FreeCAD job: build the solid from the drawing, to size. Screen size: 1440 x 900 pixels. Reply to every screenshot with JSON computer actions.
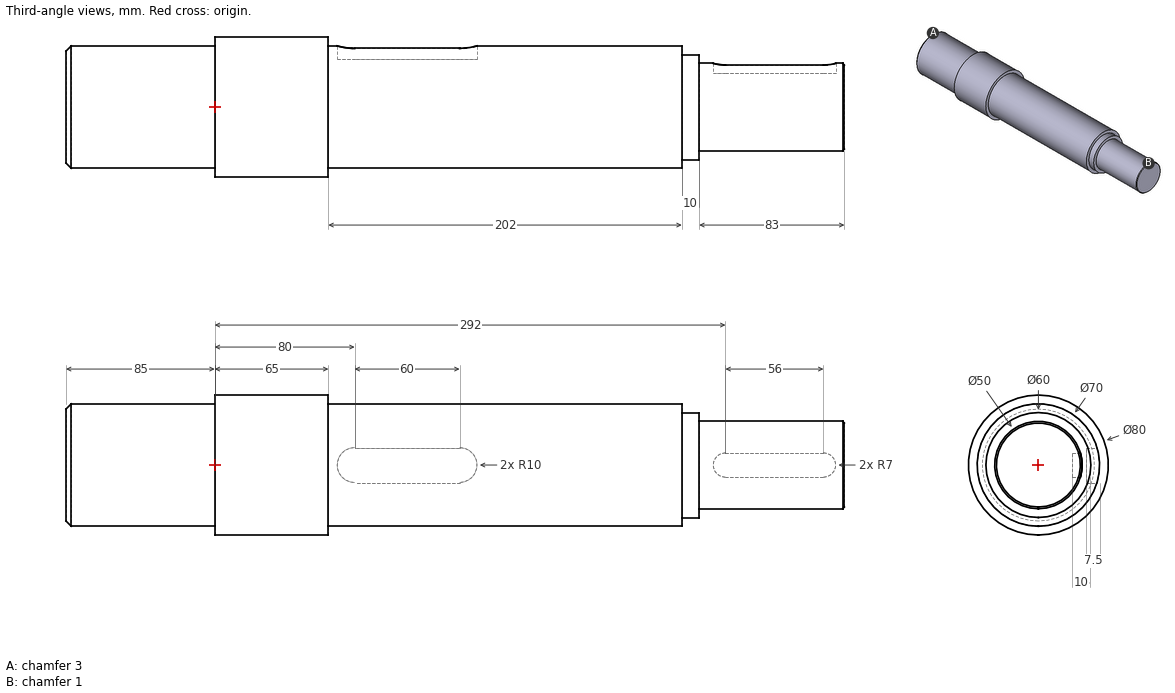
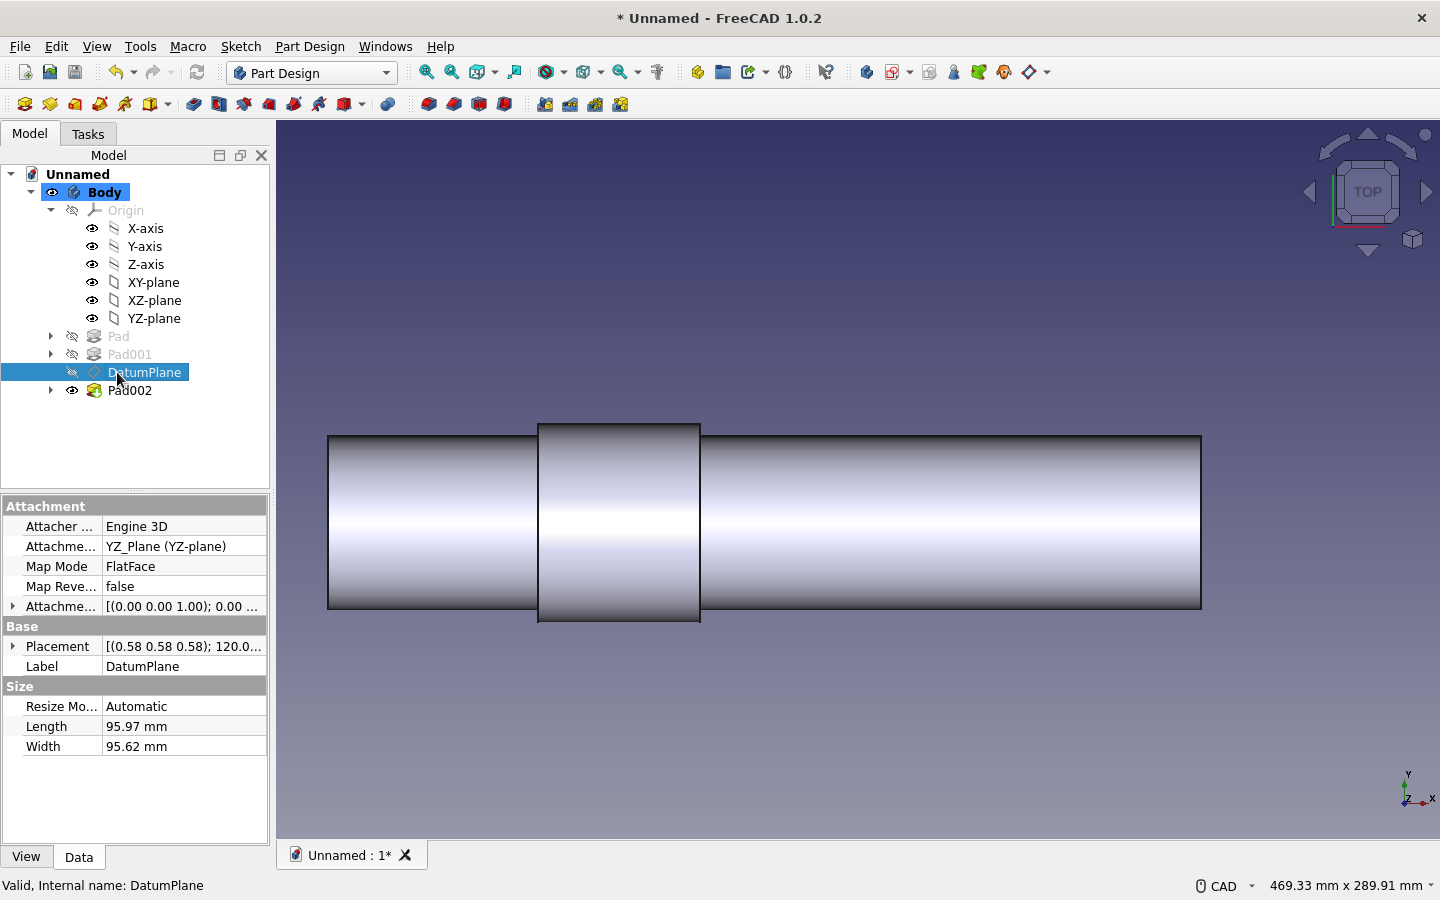
{"action": "left_click", "coordinate": [328, 592]}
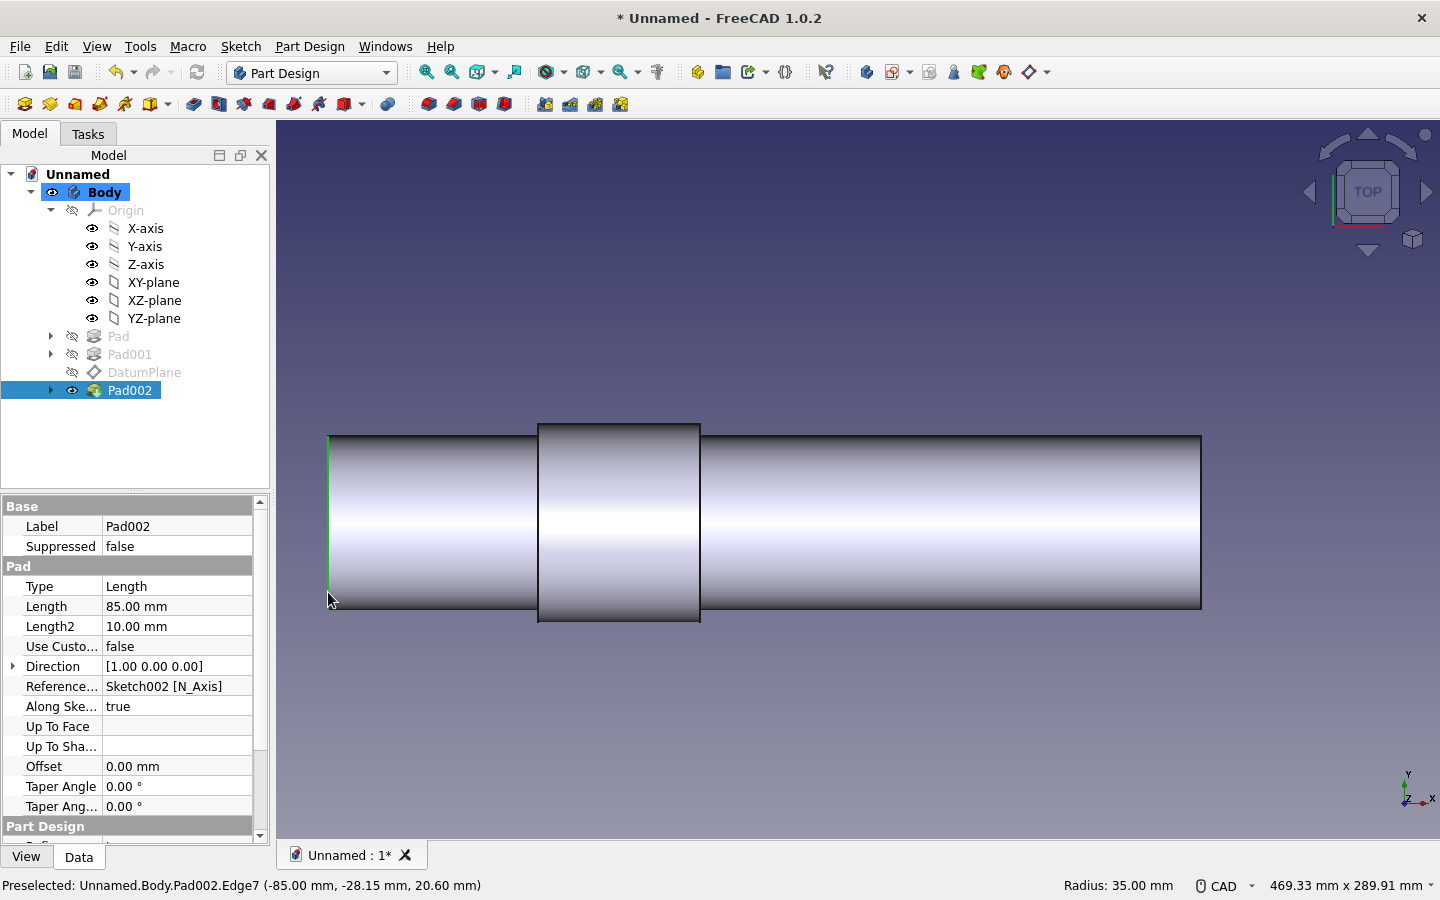
{"action": "left_click", "coordinate": [454, 104]}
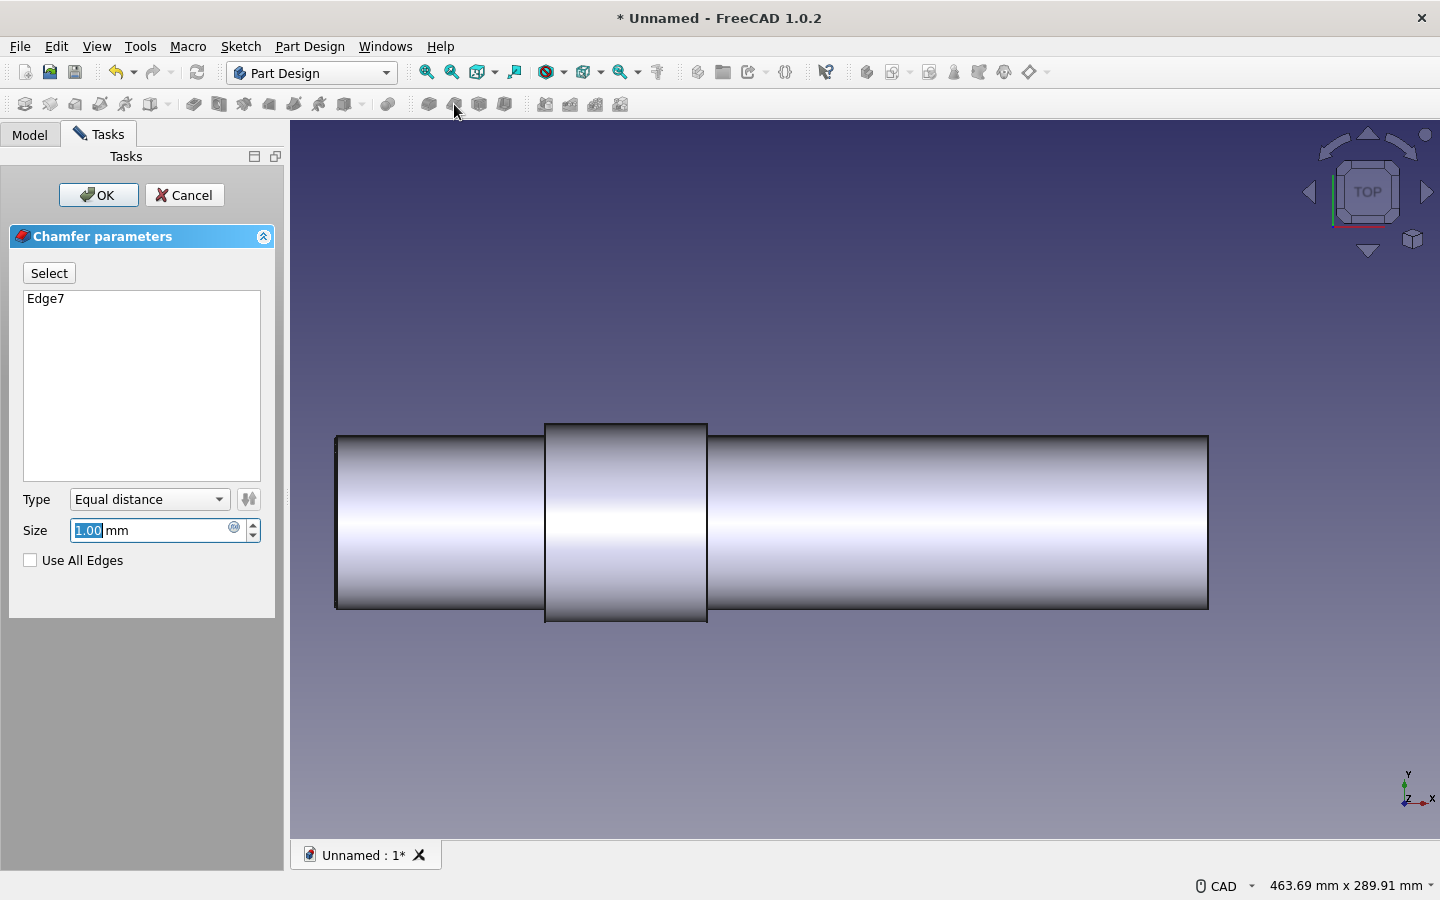
{"action": "type", "text": "3"}
{"action": "key", "text": "Tab"}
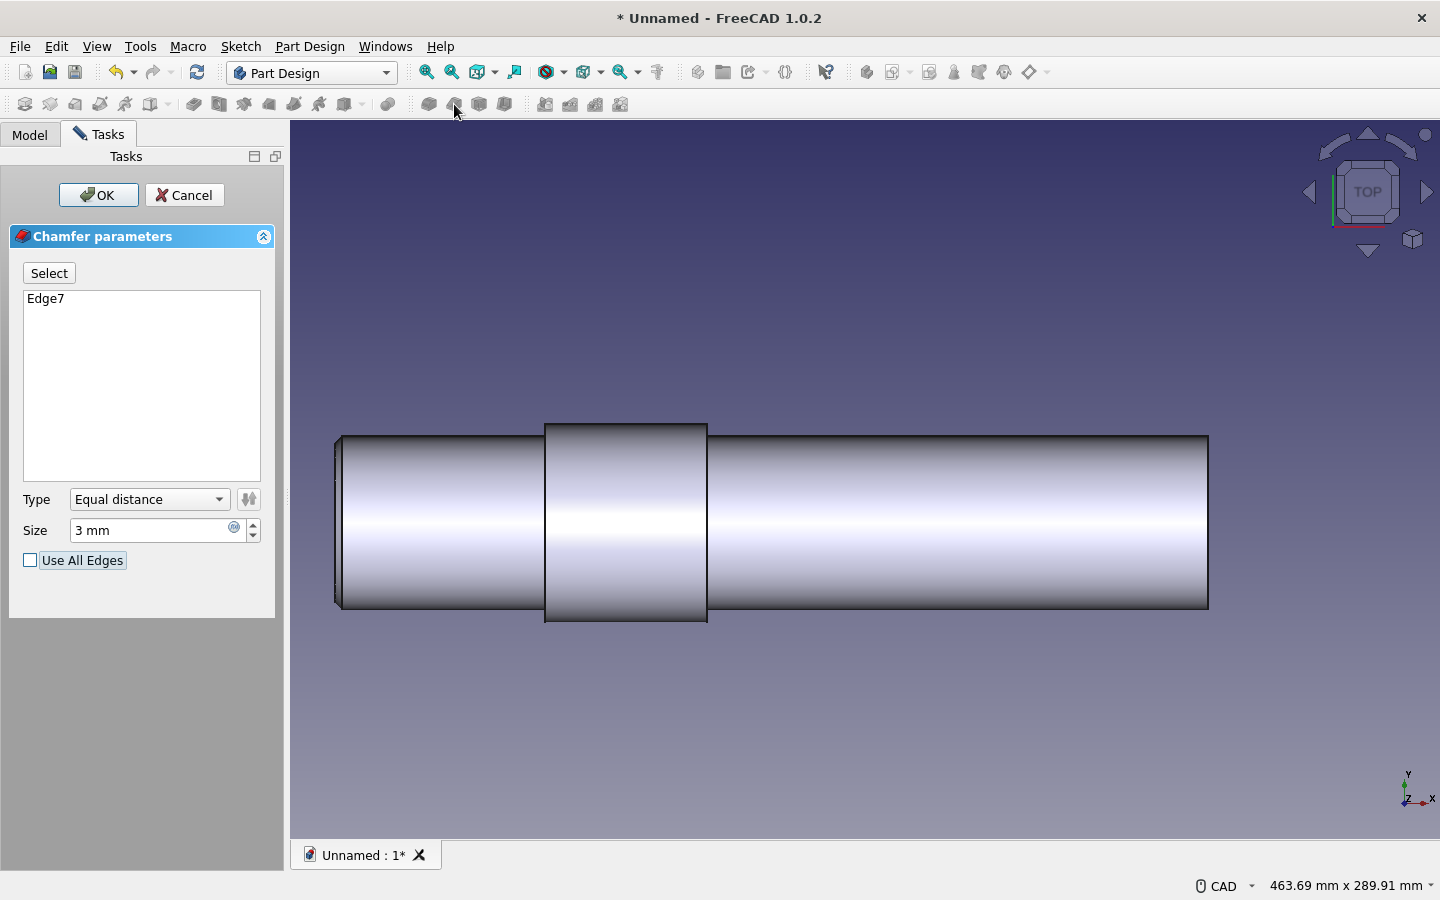
{"action": "left_click", "coordinate": [99, 195]}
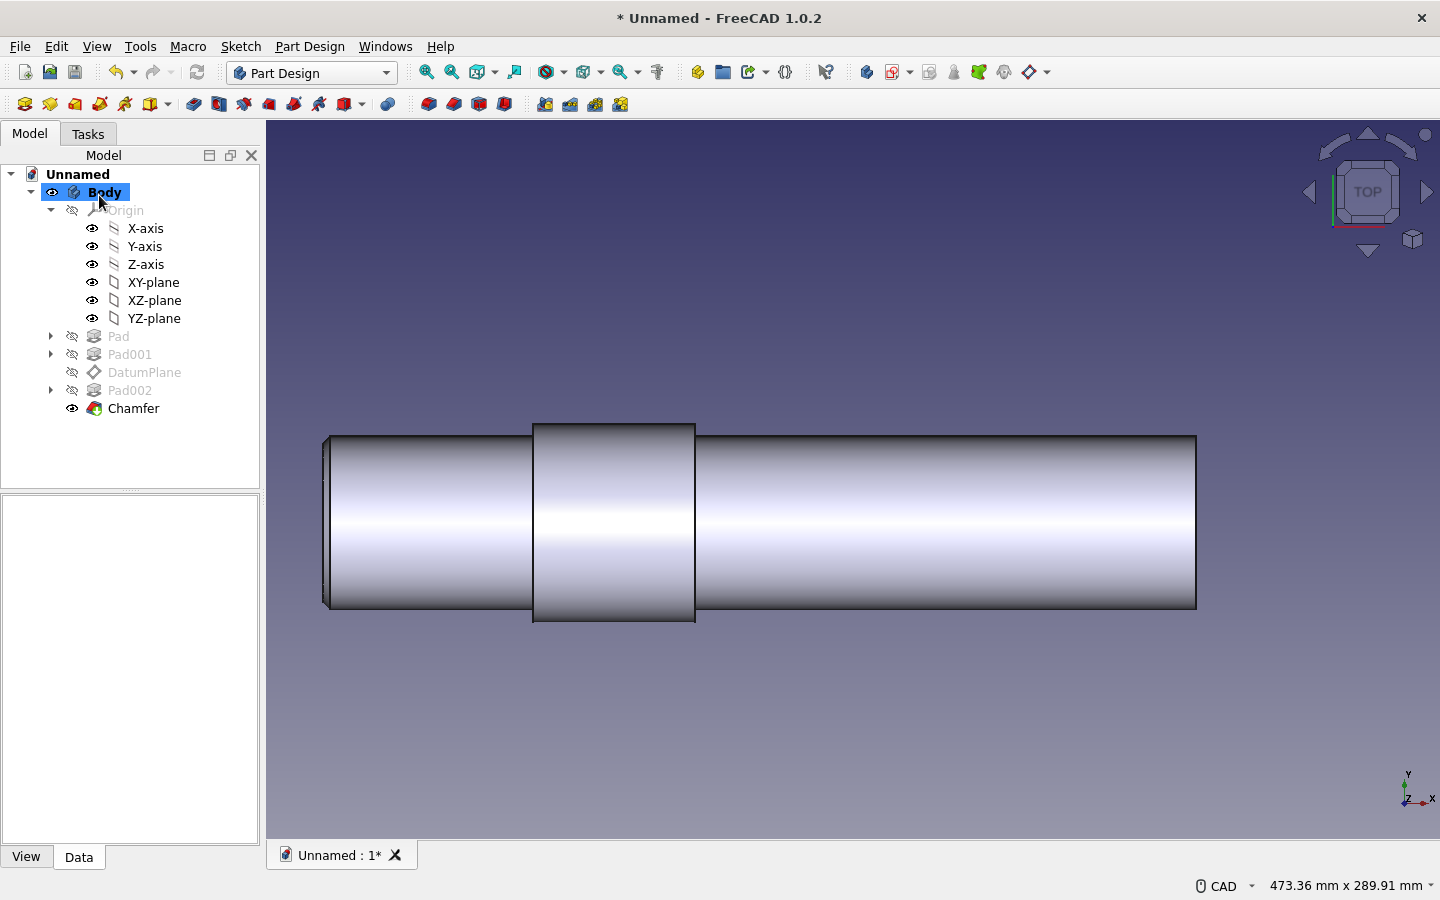
{"action": "left_click", "coordinate": [137, 300]}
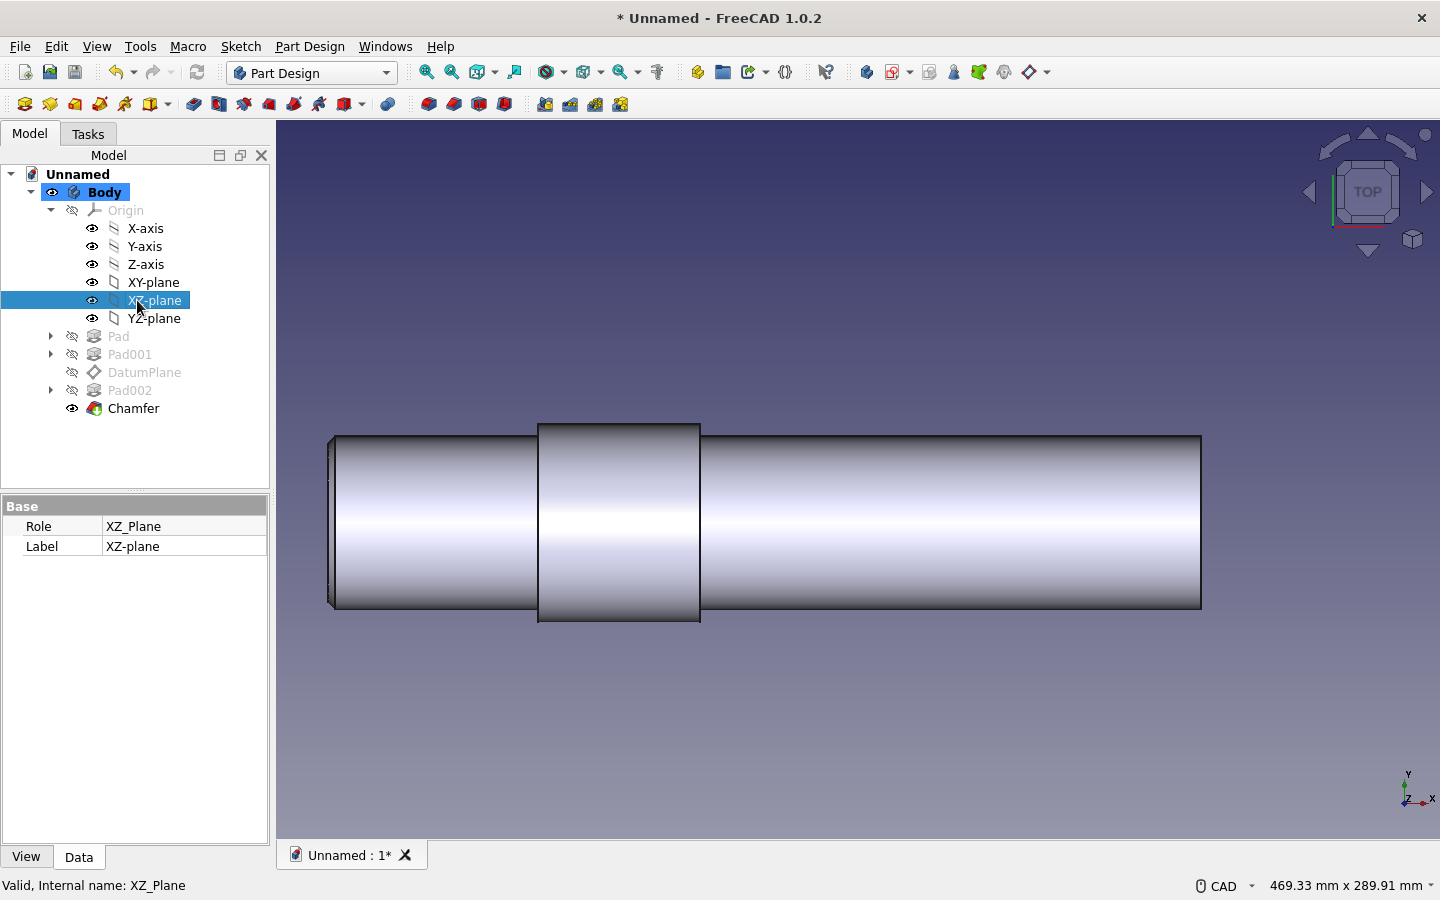
{"action": "left_click", "coordinate": [1028, 72]}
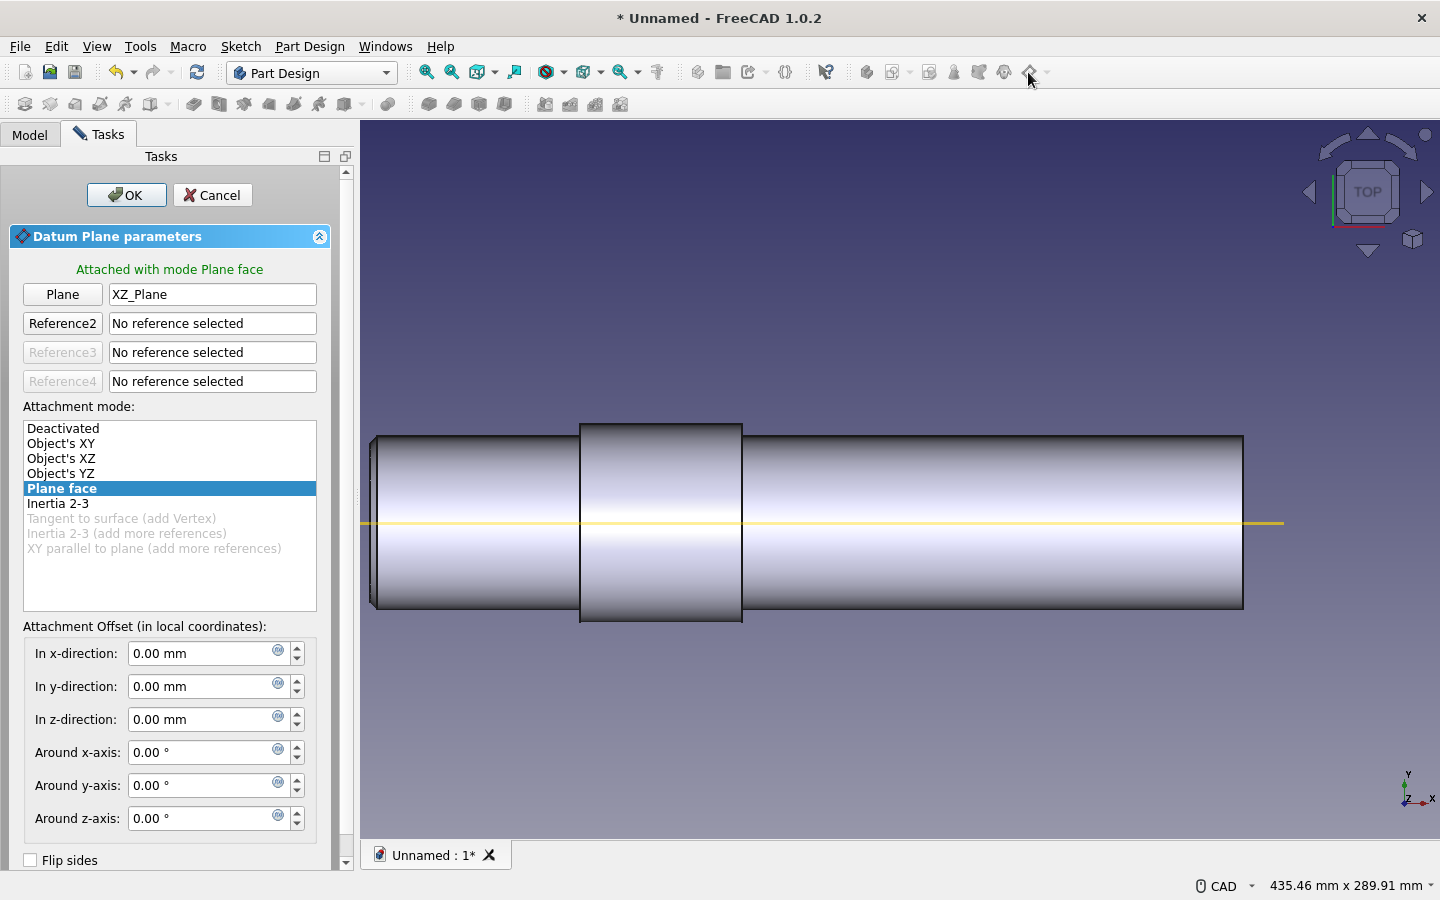
{"action": "triple_click", "coordinate": [210, 720]}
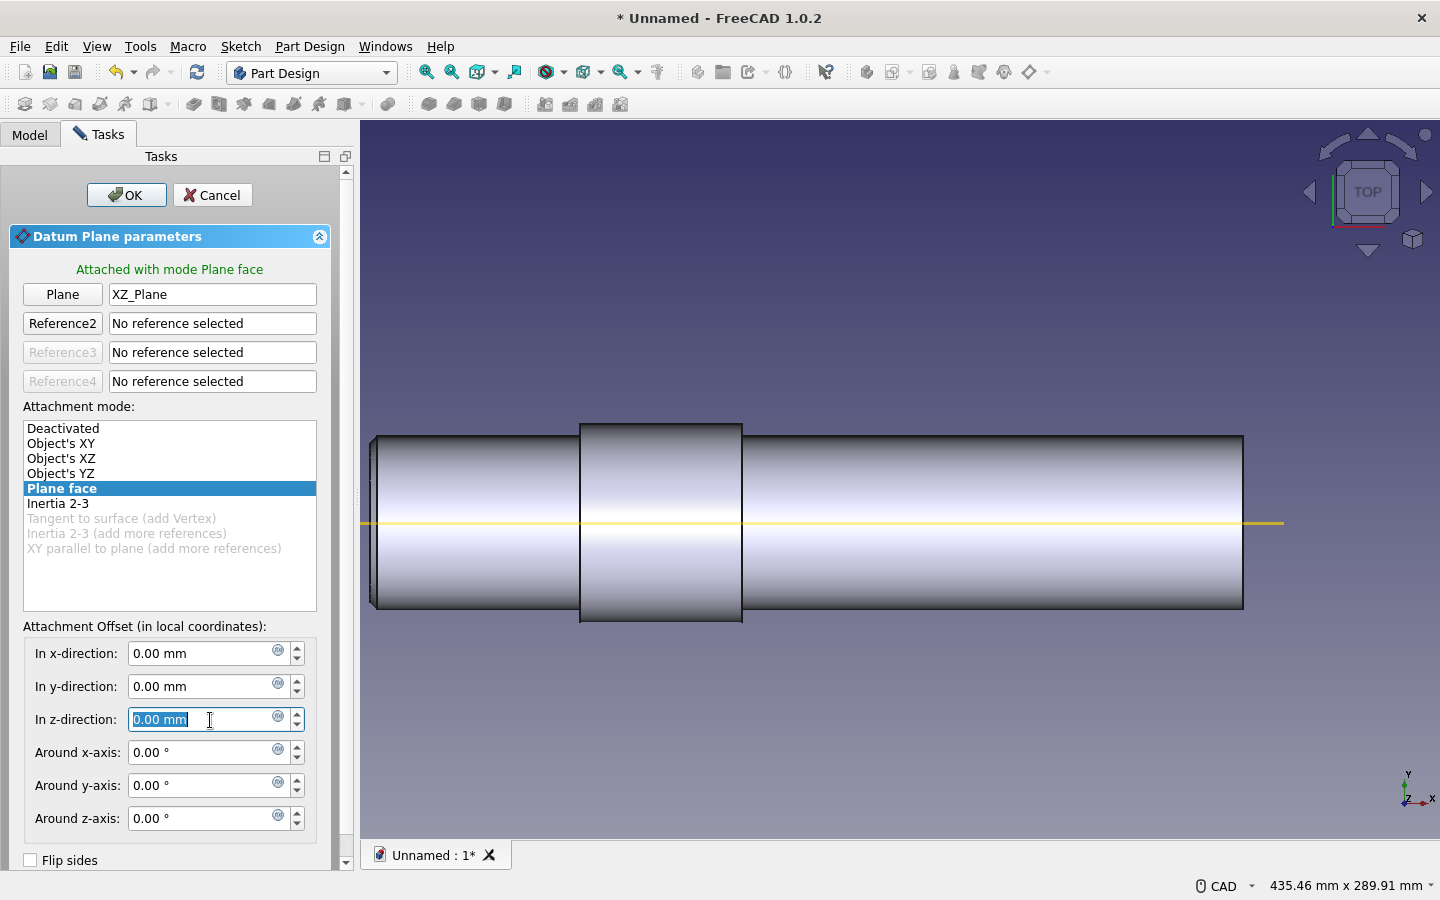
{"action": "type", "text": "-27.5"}
{"action": "key", "text": "Tab"}